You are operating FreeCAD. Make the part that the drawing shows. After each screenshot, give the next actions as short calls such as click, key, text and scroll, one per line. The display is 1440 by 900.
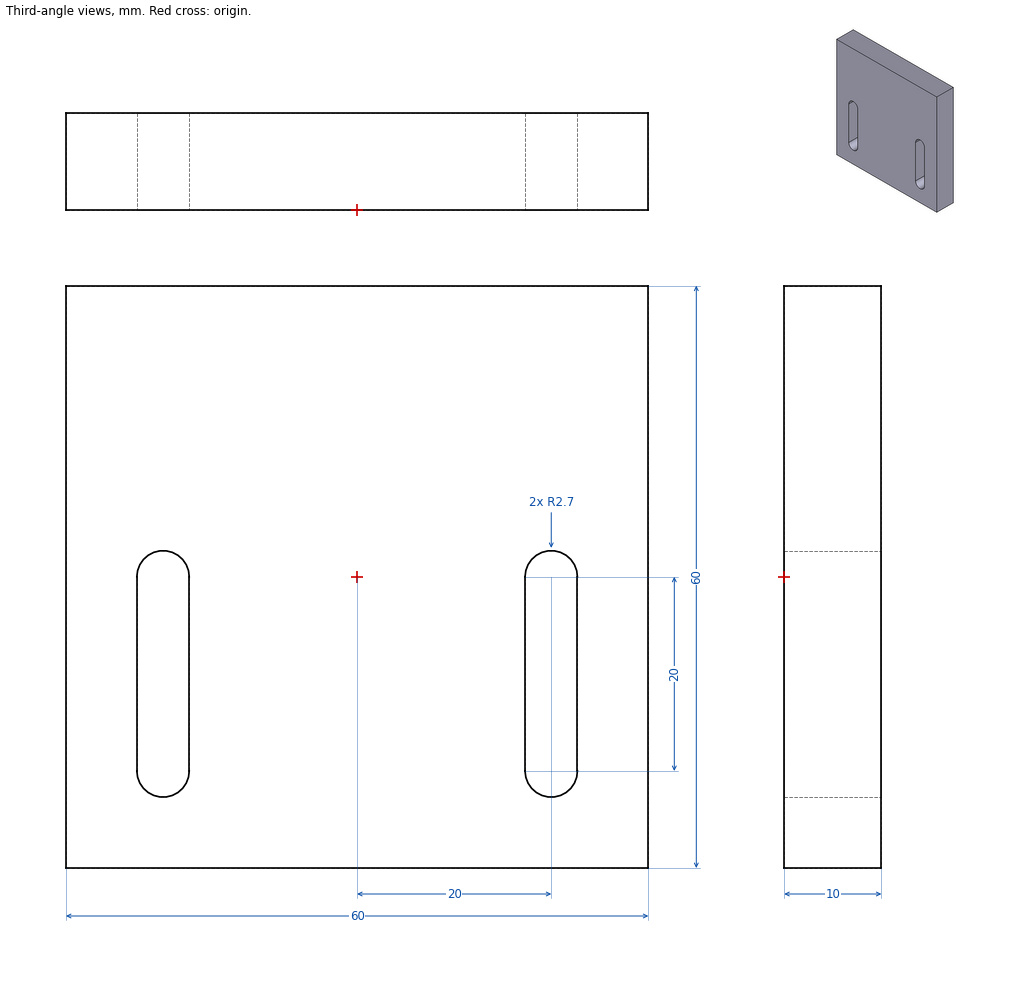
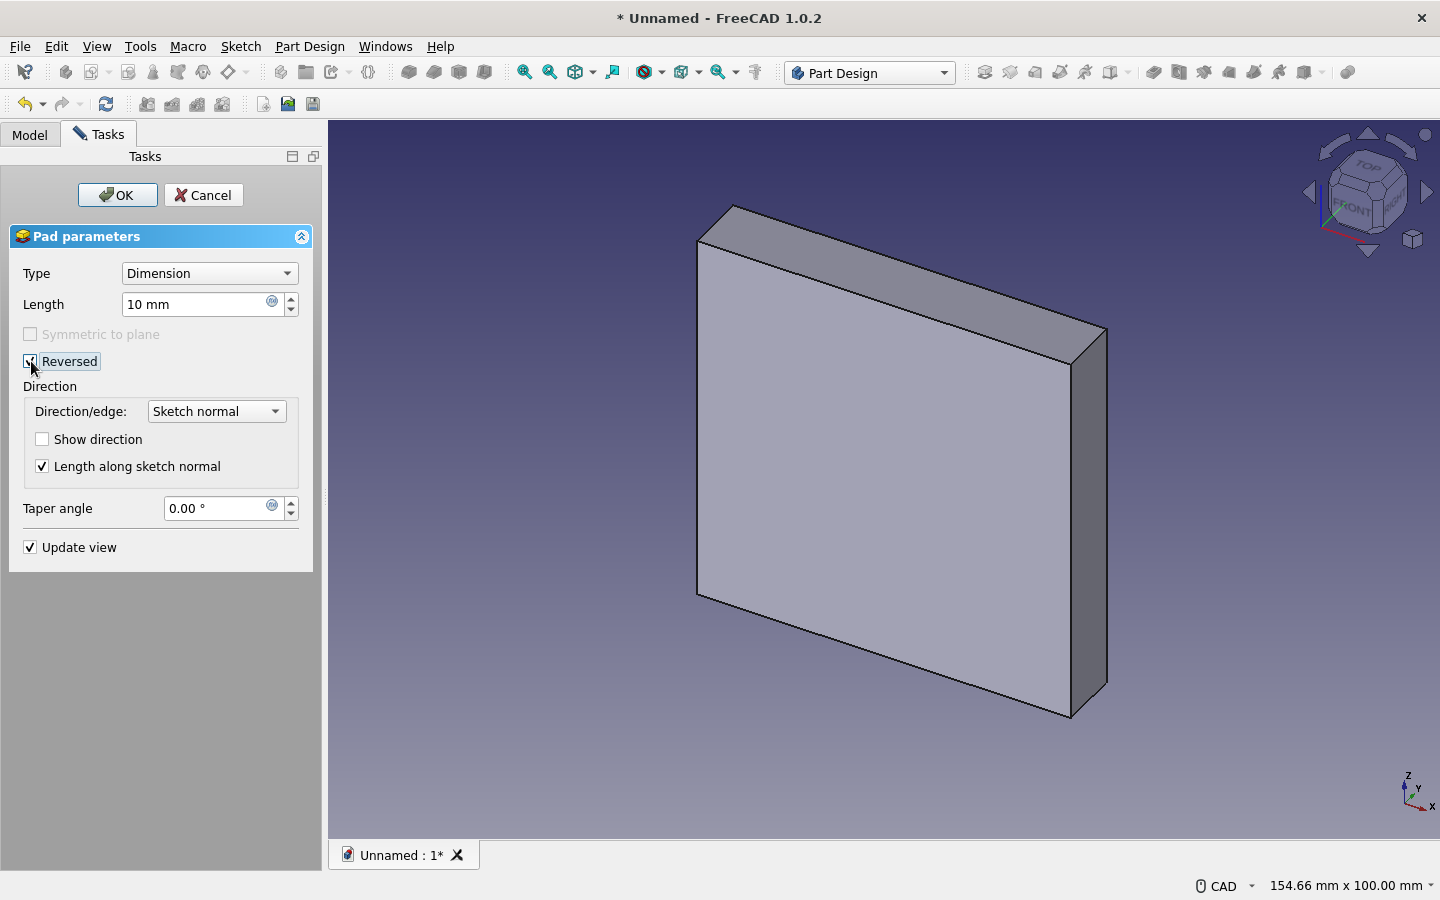
click(118, 195)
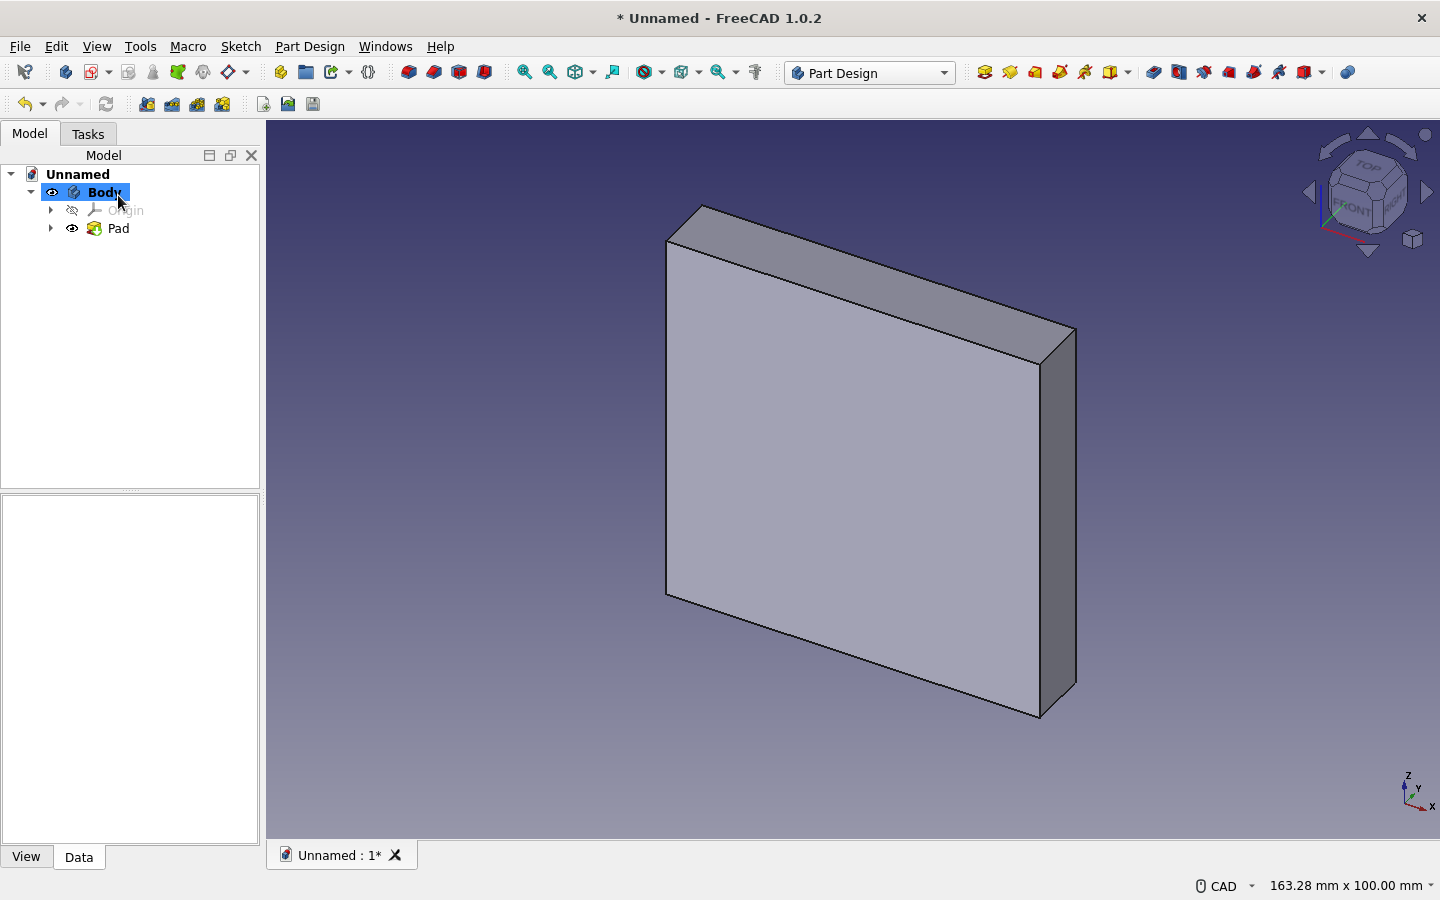
key(4)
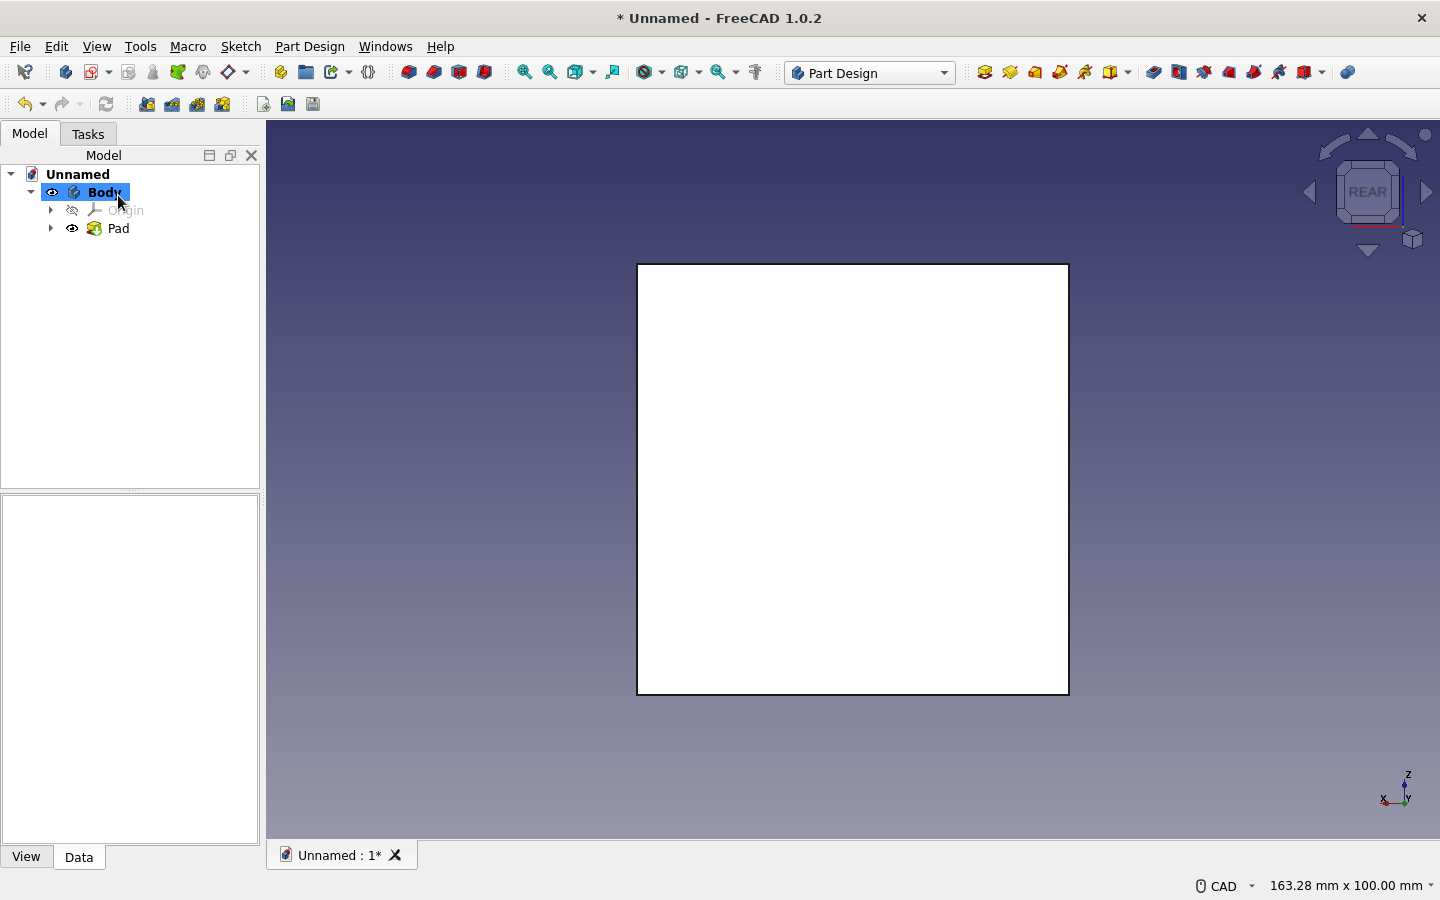
click(853, 478)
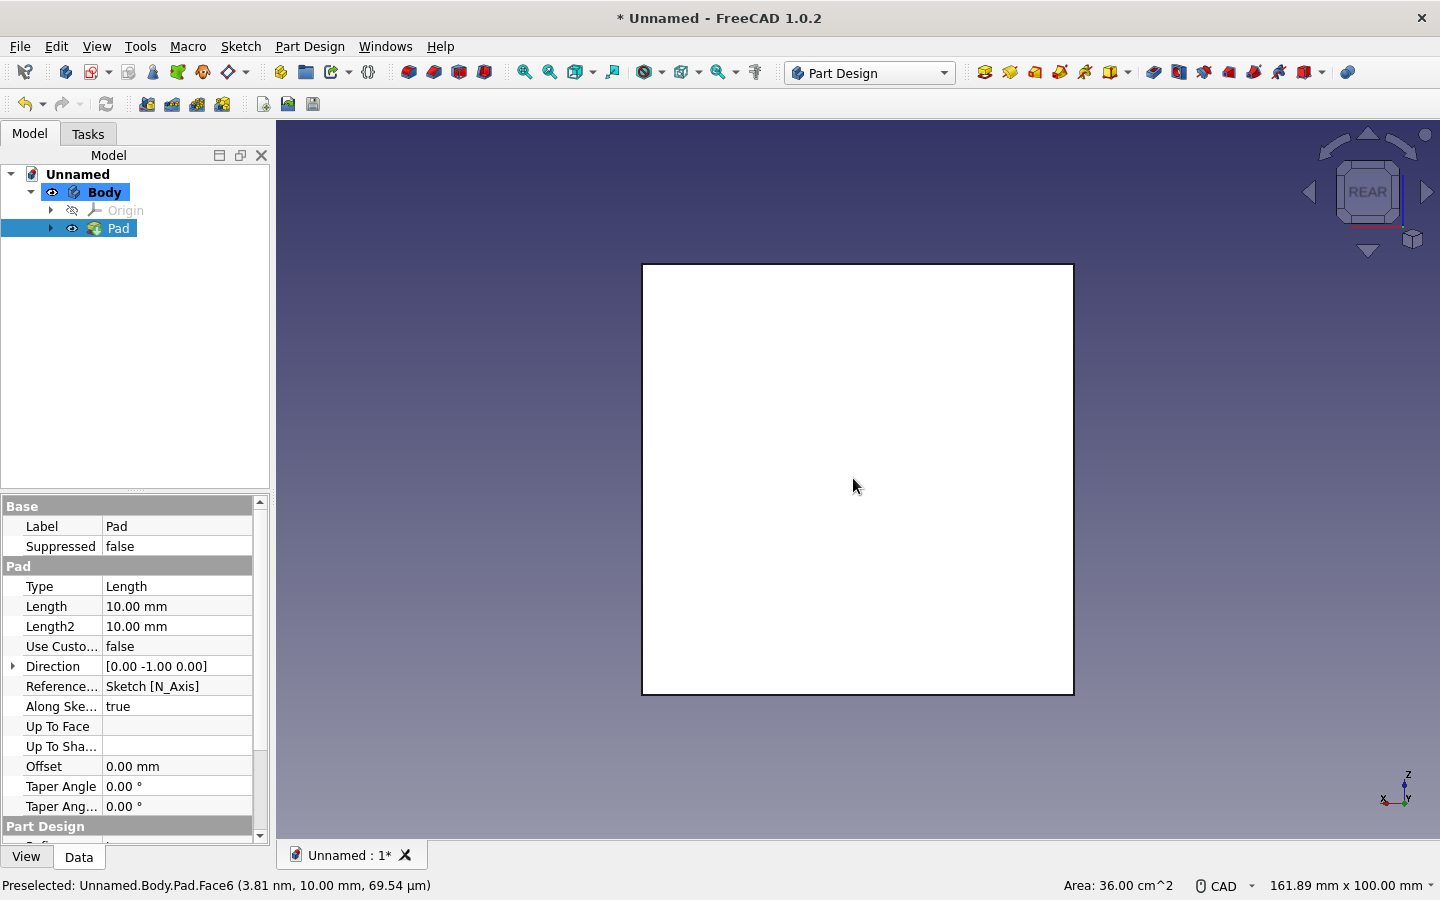
click(90, 72)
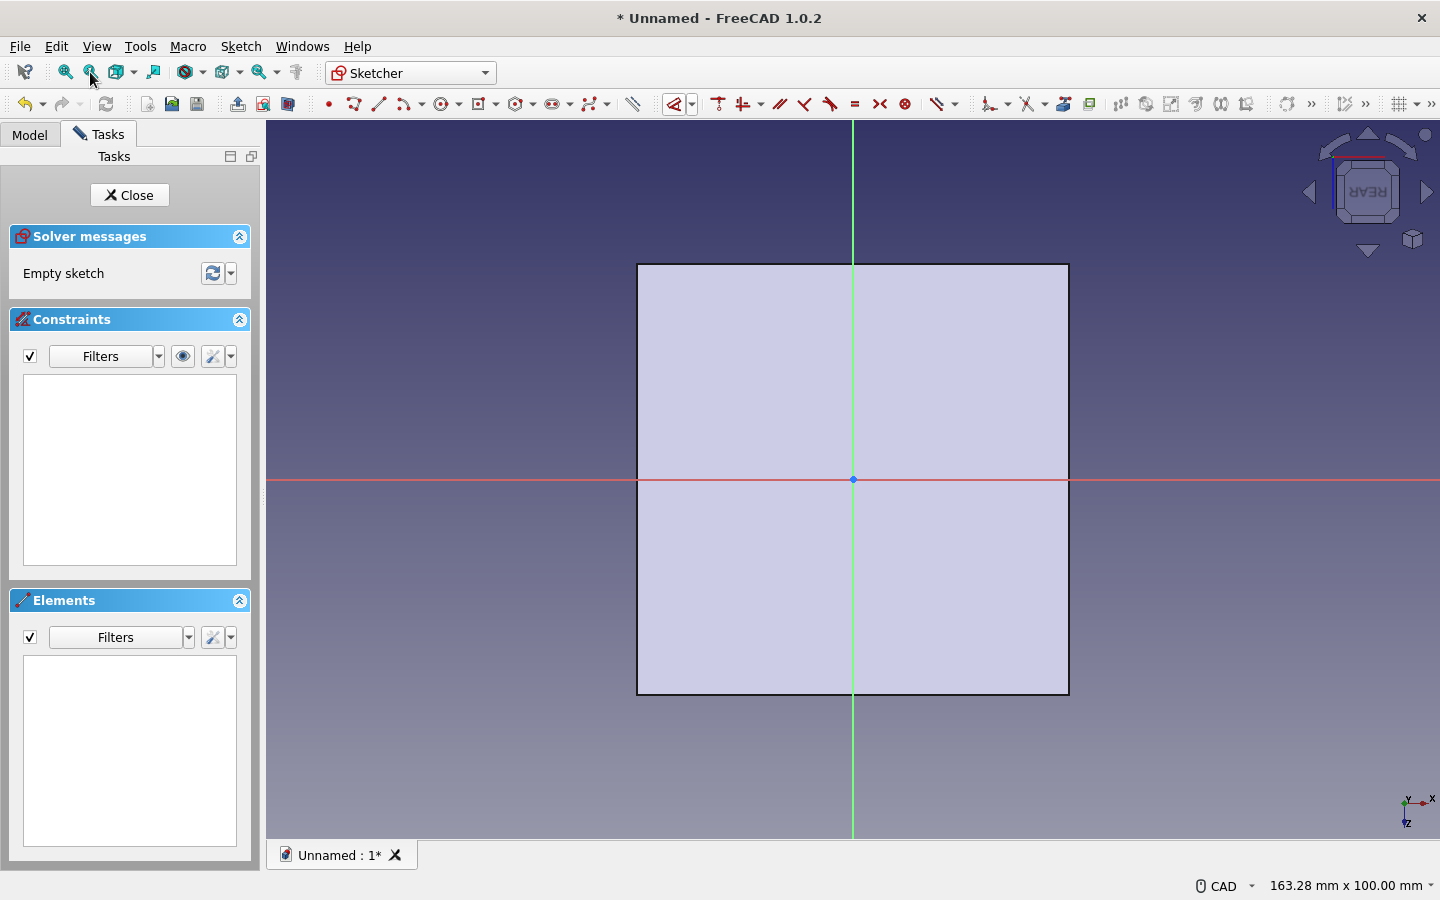
scroll(1022, 366, up, 5)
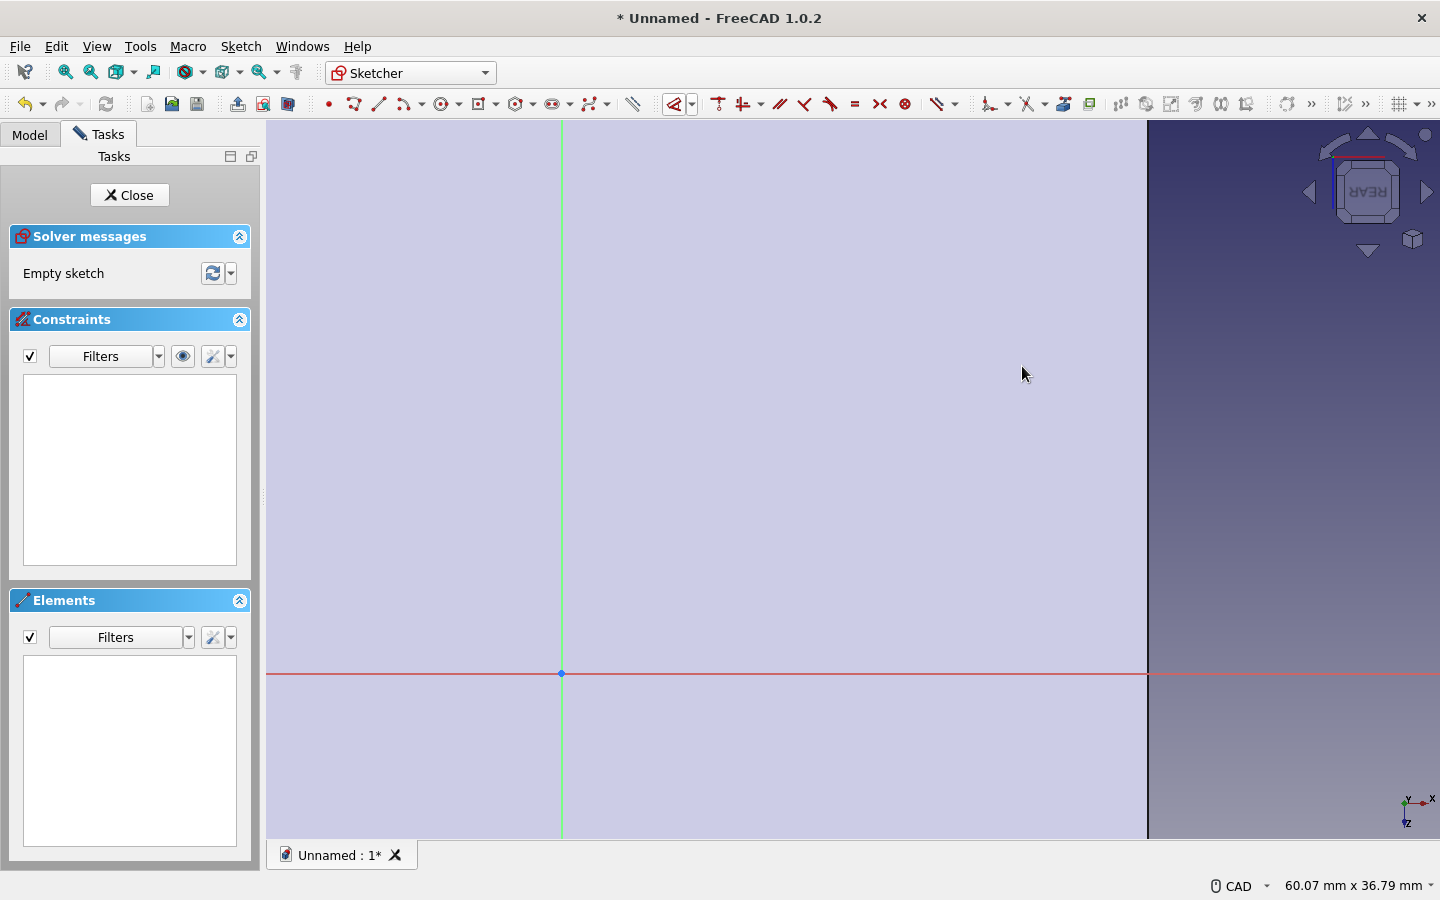
click(552, 104)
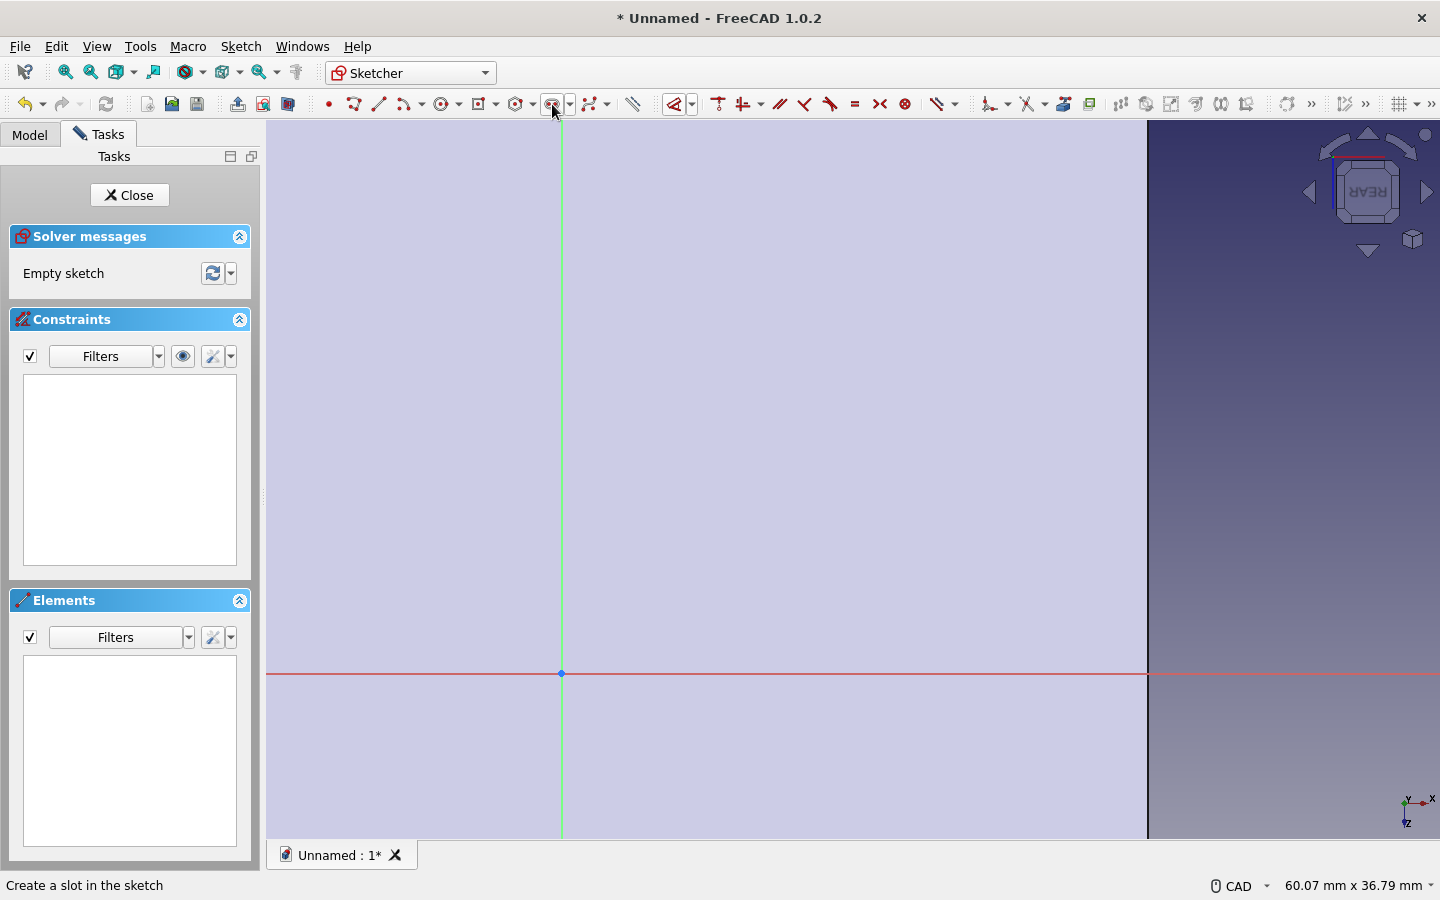
click(952, 674)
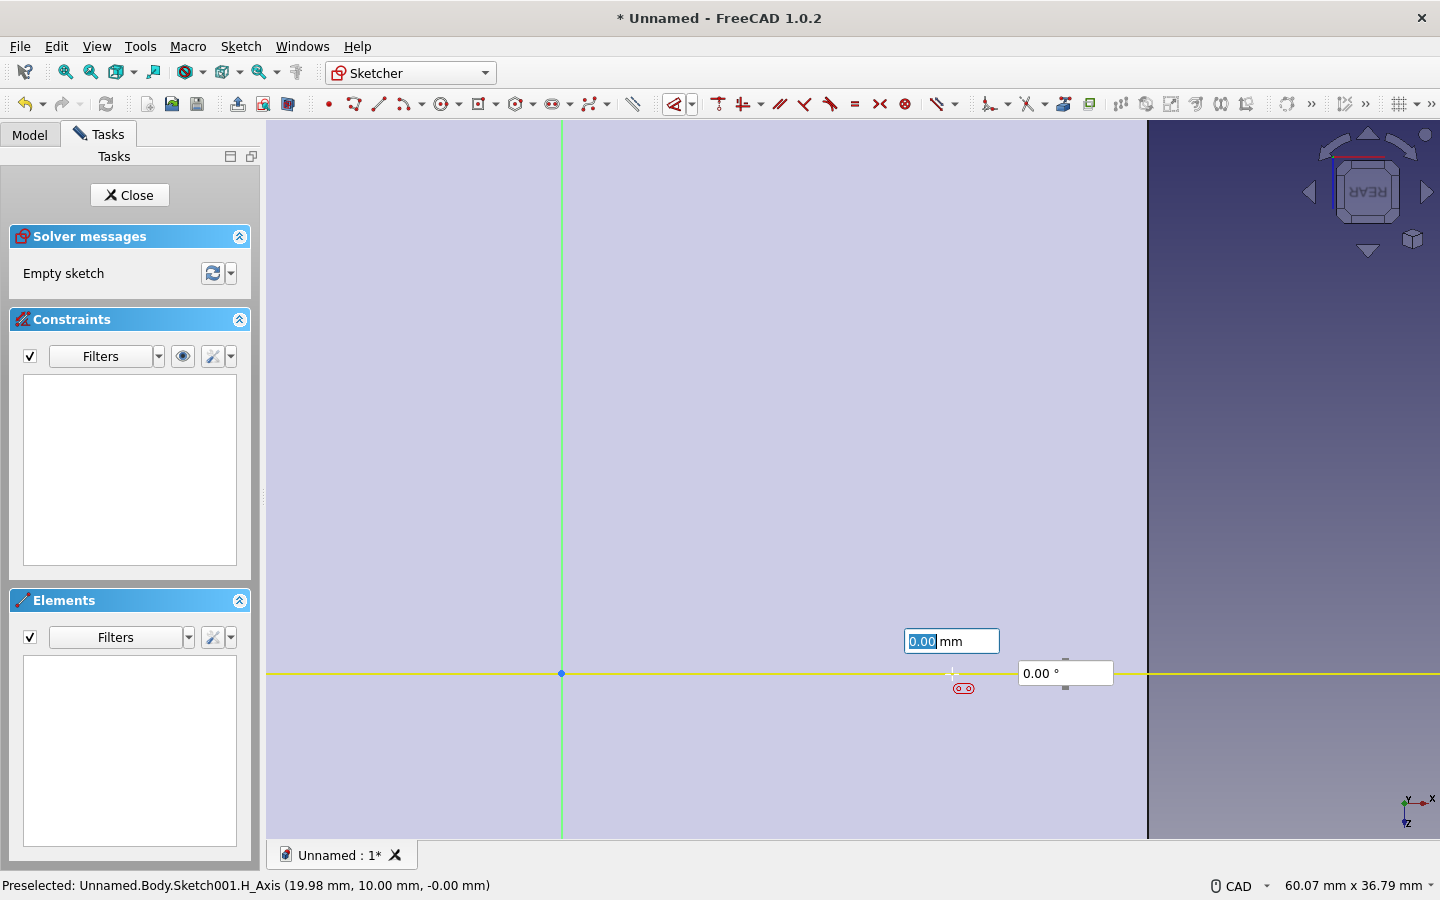
click(952, 283)